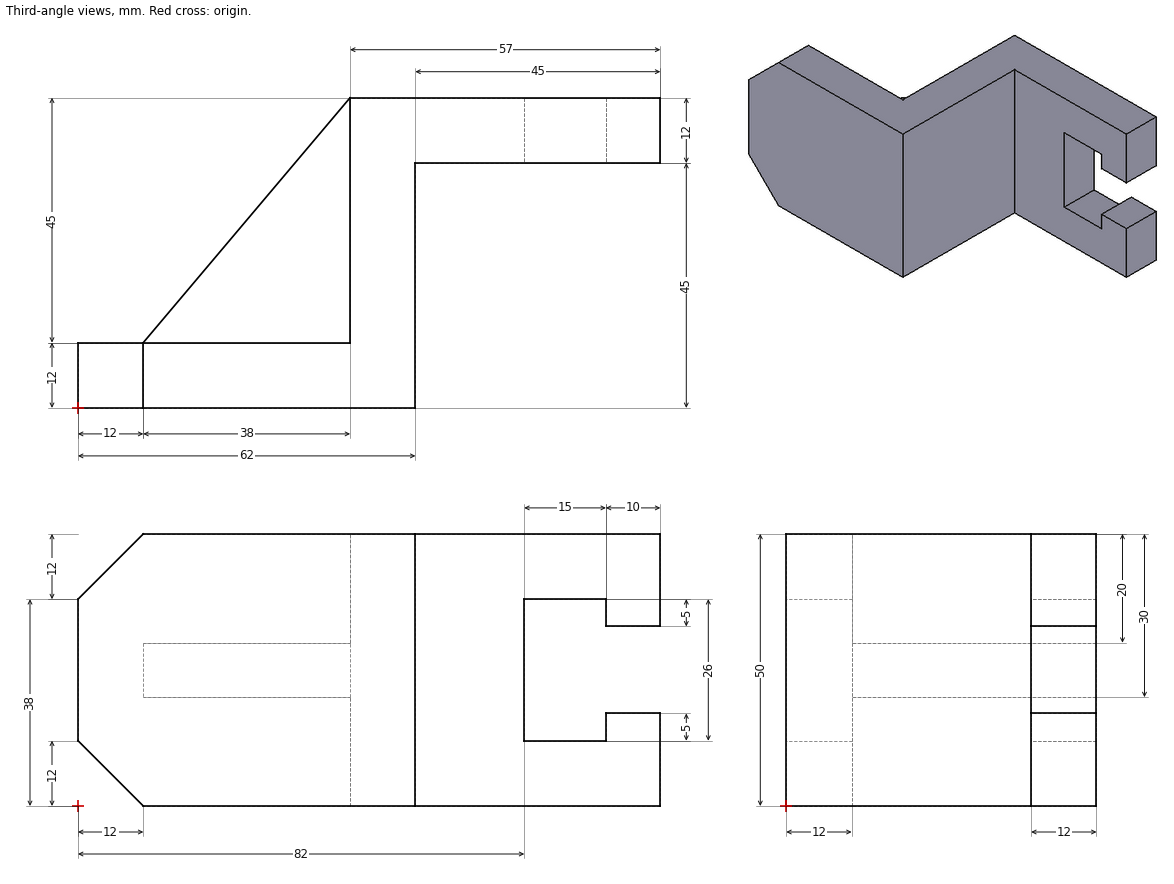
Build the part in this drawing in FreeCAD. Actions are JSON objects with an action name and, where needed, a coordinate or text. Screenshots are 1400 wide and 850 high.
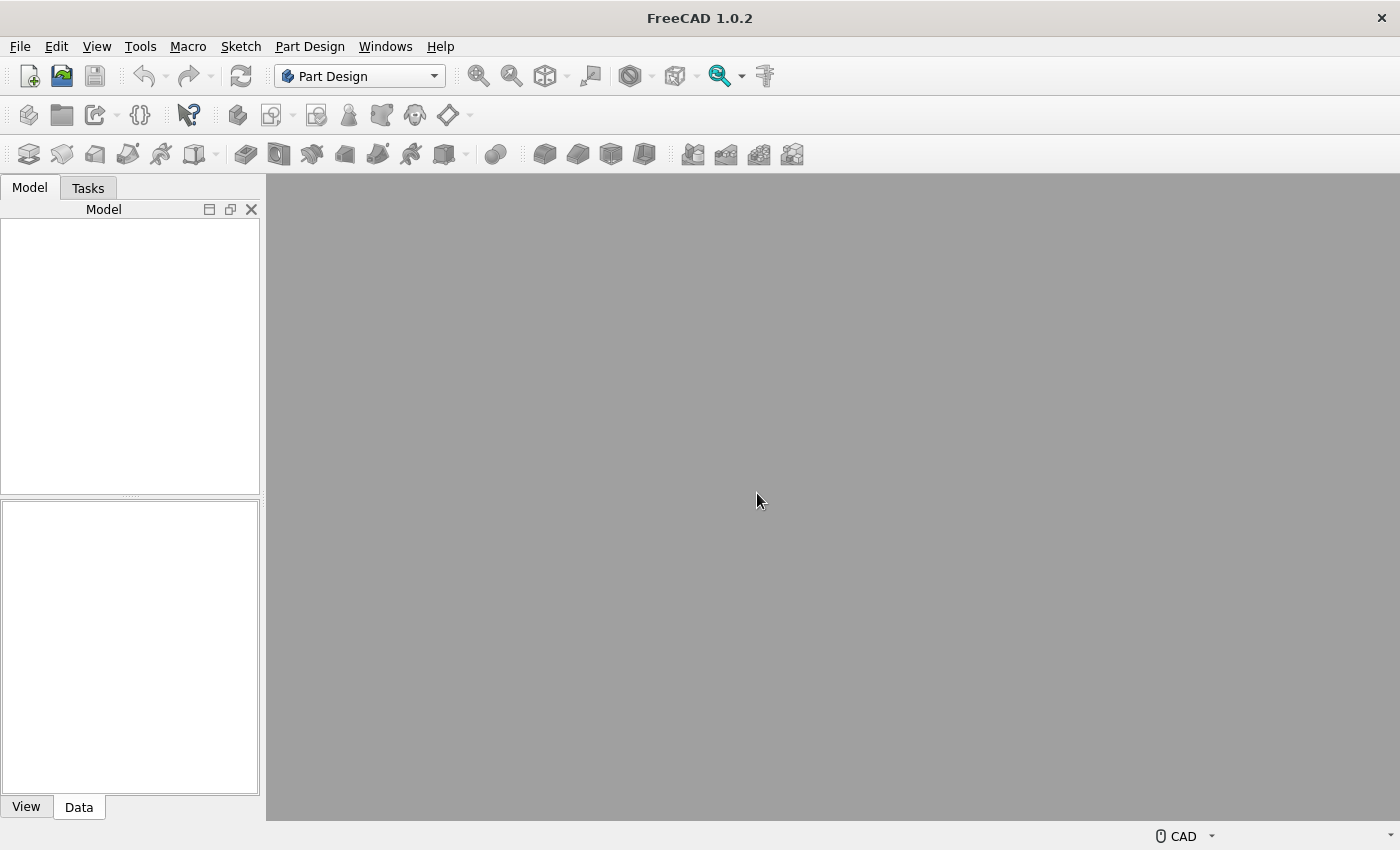
{"action": "left_click", "coordinate": [29, 76]}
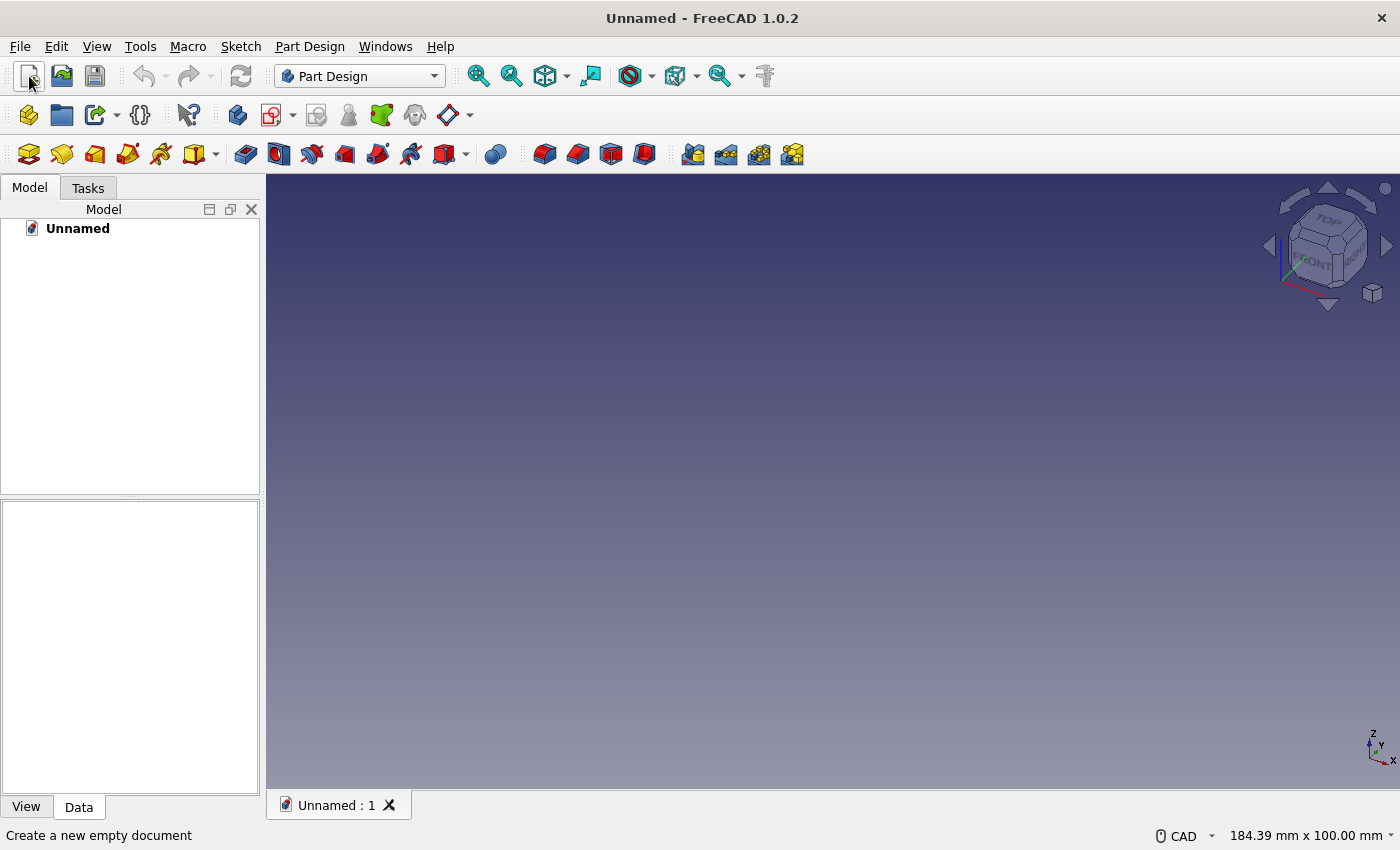
{"action": "left_click", "coordinate": [270, 116]}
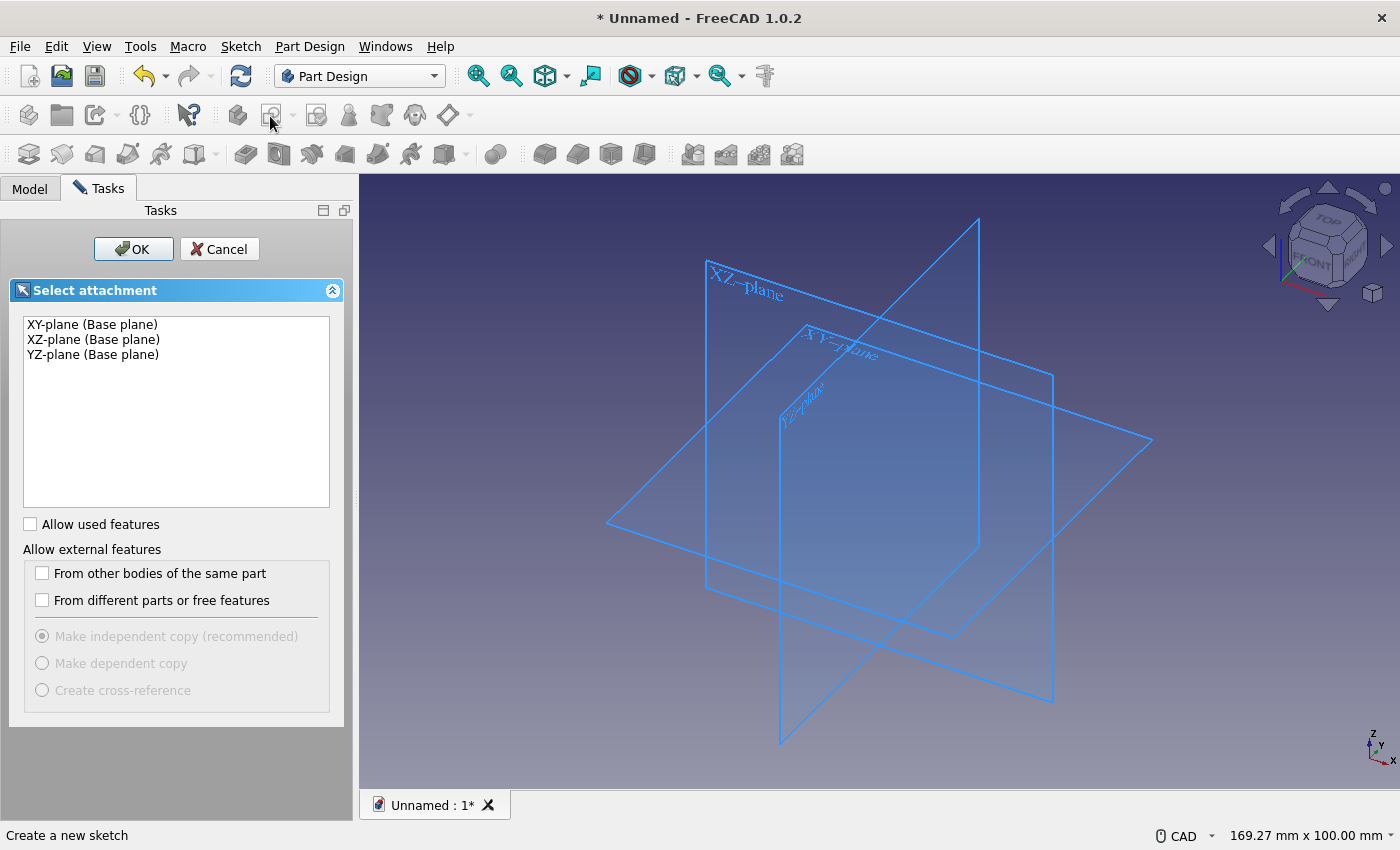
{"action": "left_click", "coordinate": [84, 324]}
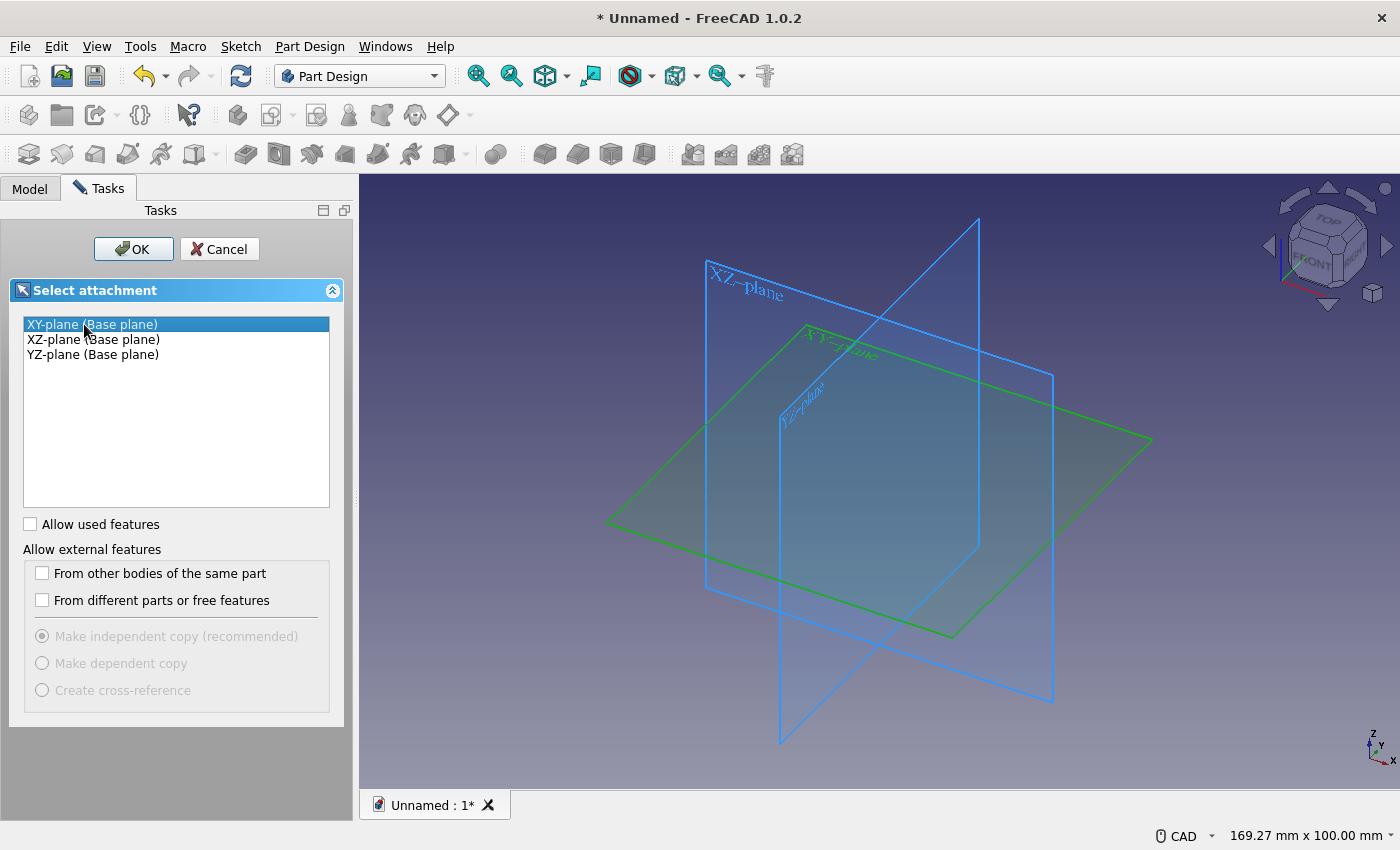
{"action": "left_click", "coordinate": [134, 249]}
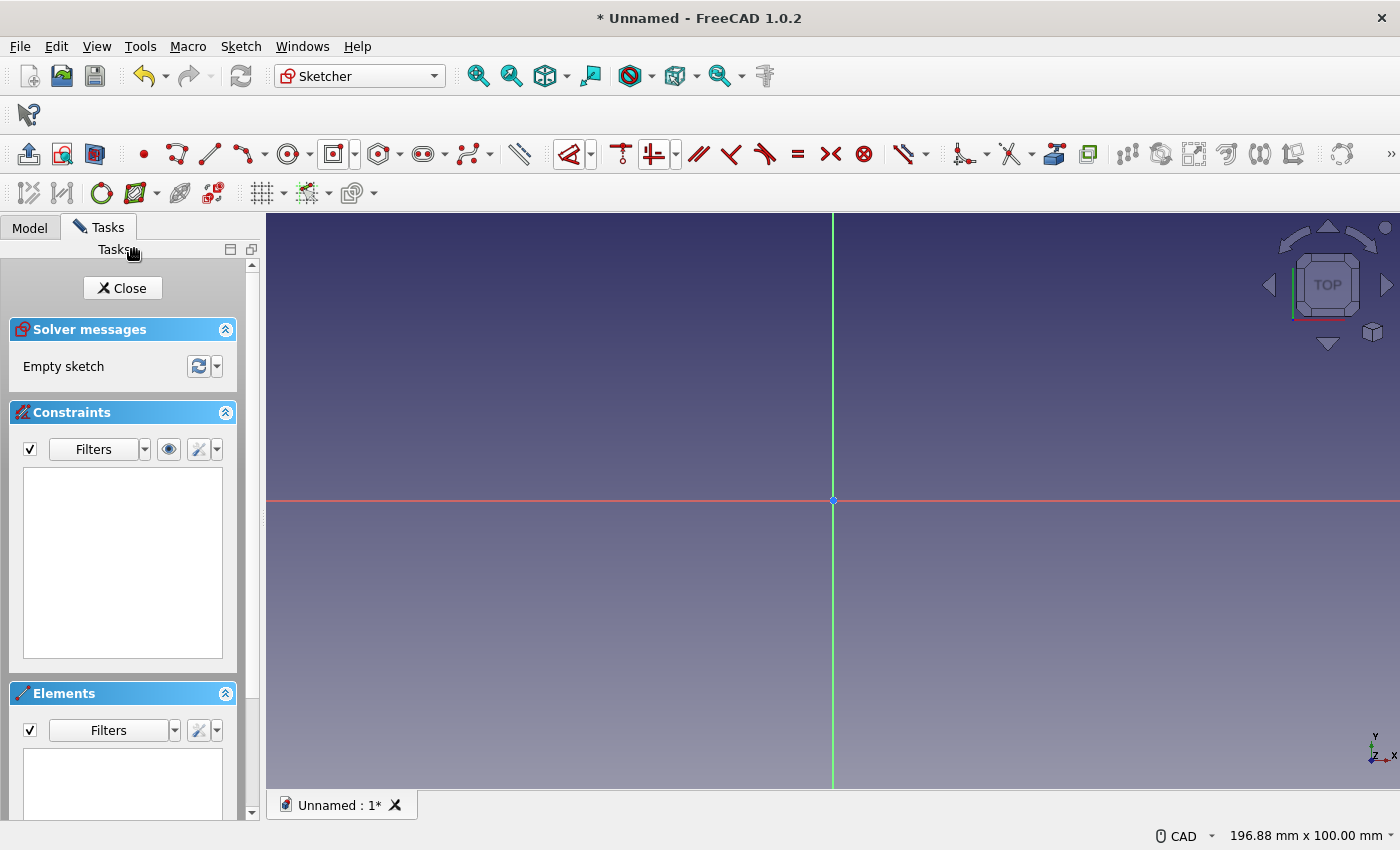
{"action": "scroll", "coordinate": [294, 761], "scroll_direction": "down", "scroll_amount": 2}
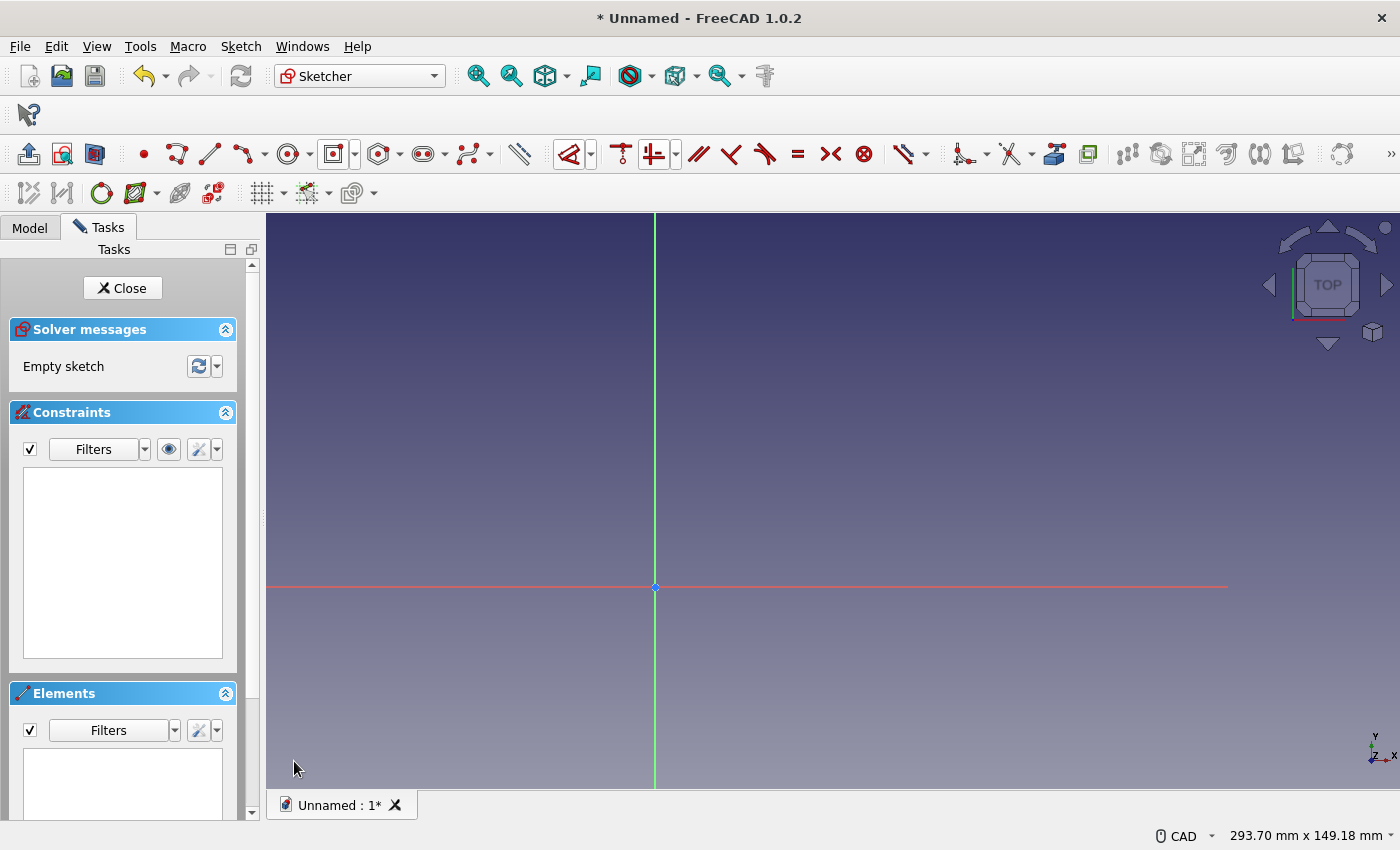
{"action": "scroll", "coordinate": [1060, 428], "scroll_direction": "up", "scroll_amount": 2}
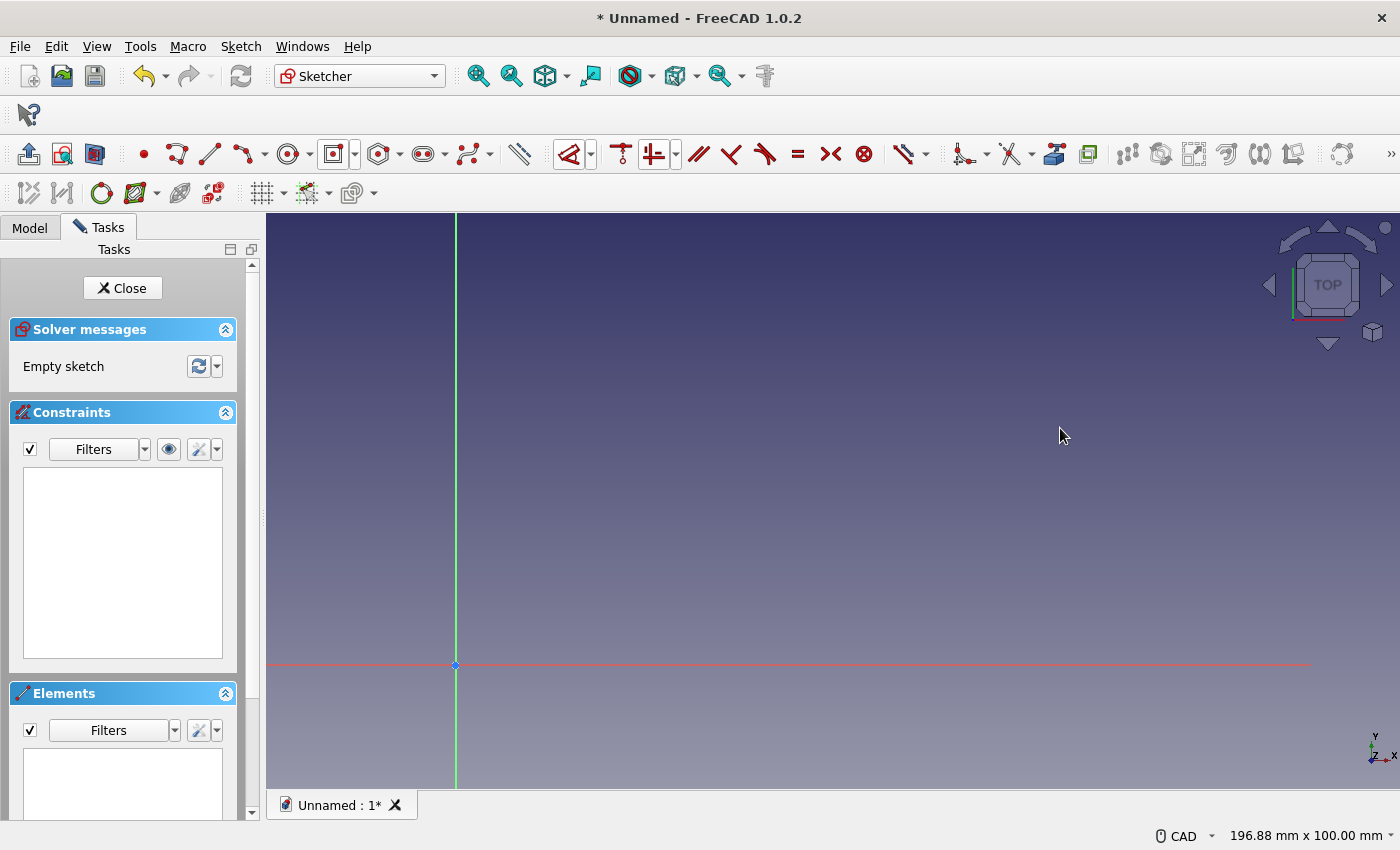
{"action": "left_click", "coordinate": [177, 154]}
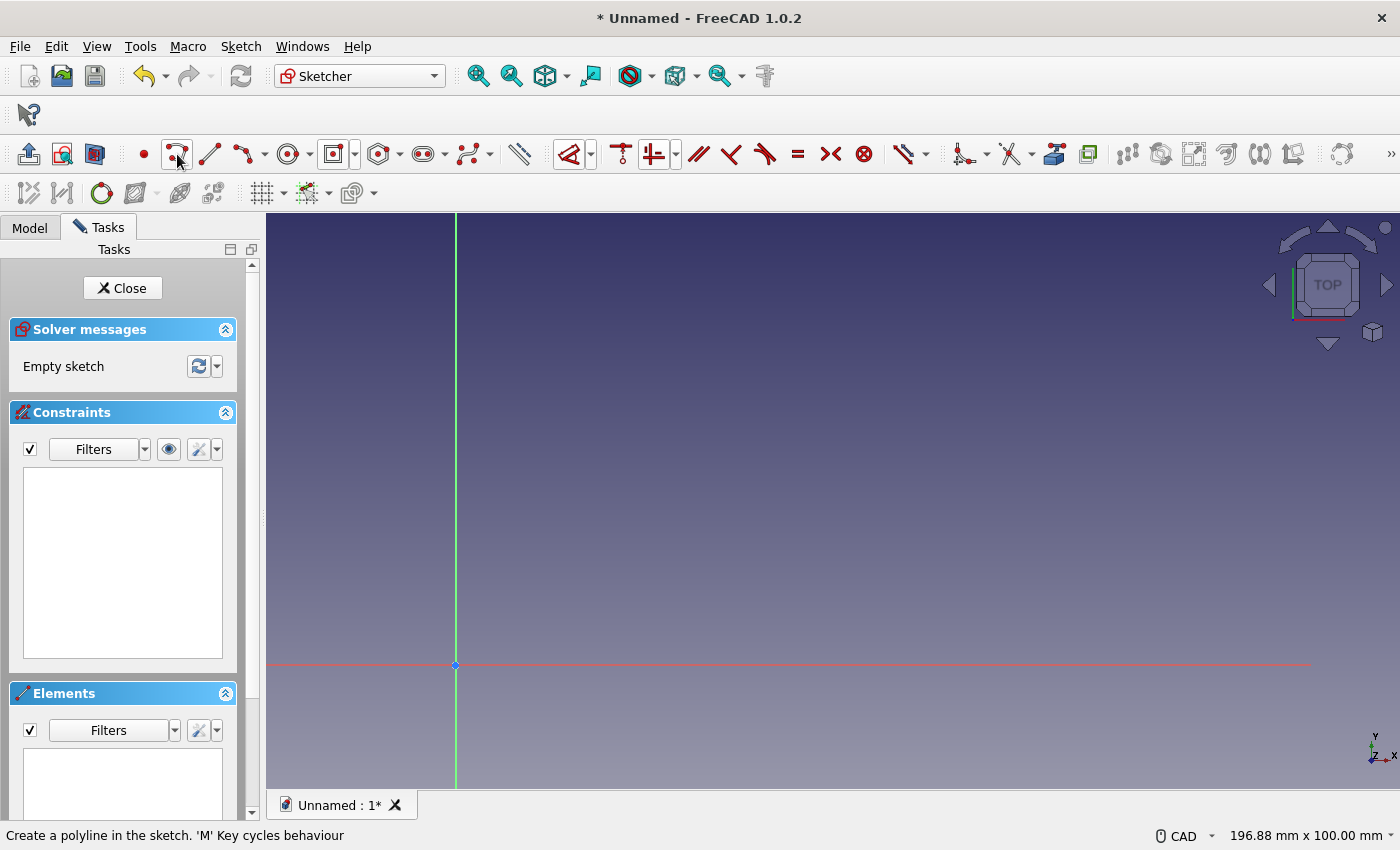
{"action": "left_click", "coordinate": [456, 665]}
{"action": "left_click", "coordinate": [813, 656]}
{"action": "left_click", "coordinate": [813, 406]}
{"action": "left_click", "coordinate": [1072, 406]}
{"action": "left_click", "coordinate": [1072, 337]}
{"action": "left_click", "coordinate": [744, 337]}
{"action": "left_click", "coordinate": [744, 596]}
{"action": "left_click", "coordinate": [465, 596]}
{"action": "left_click", "coordinate": [456, 665]}
{"action": "key", "text": "Escape"}
{"action": "key", "text": "Escape"}